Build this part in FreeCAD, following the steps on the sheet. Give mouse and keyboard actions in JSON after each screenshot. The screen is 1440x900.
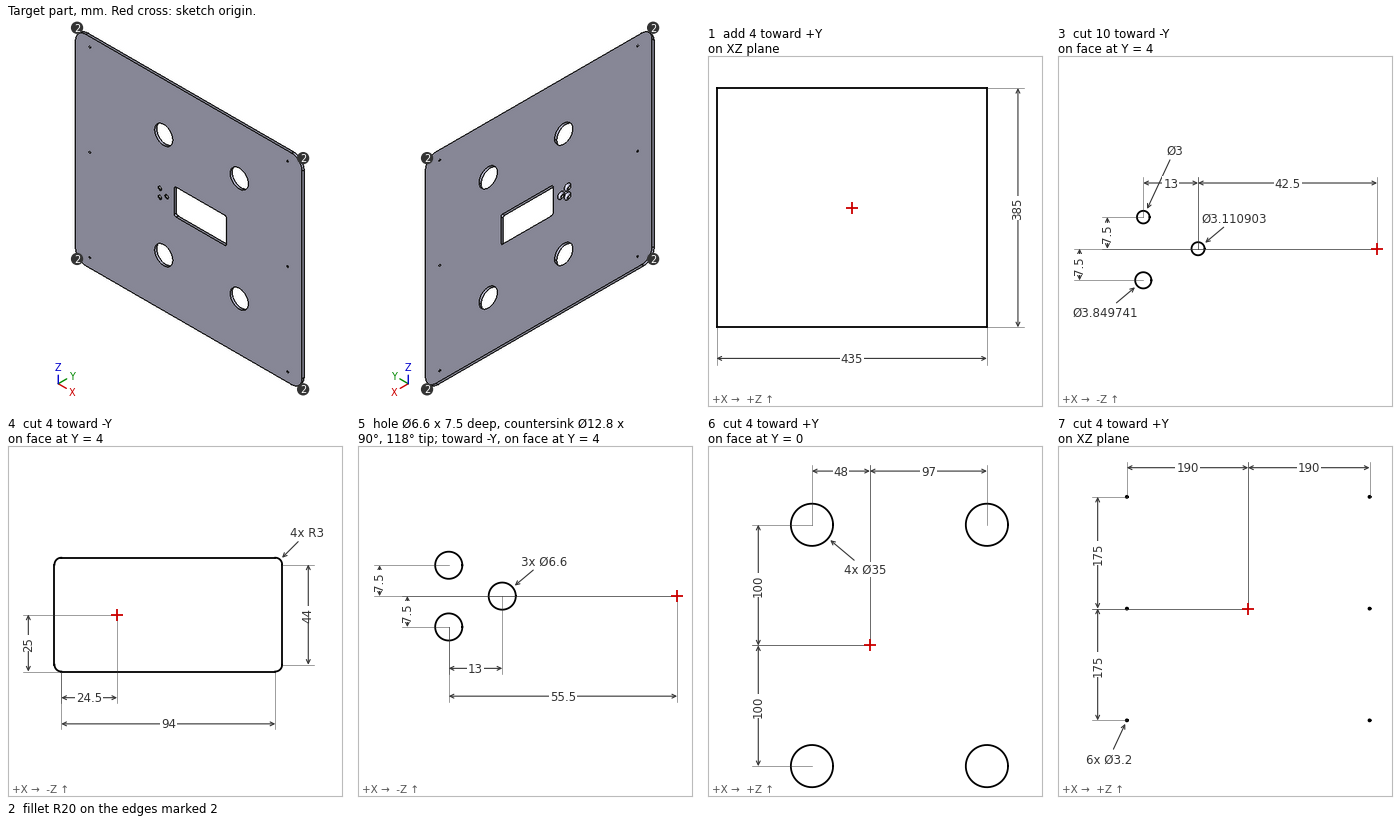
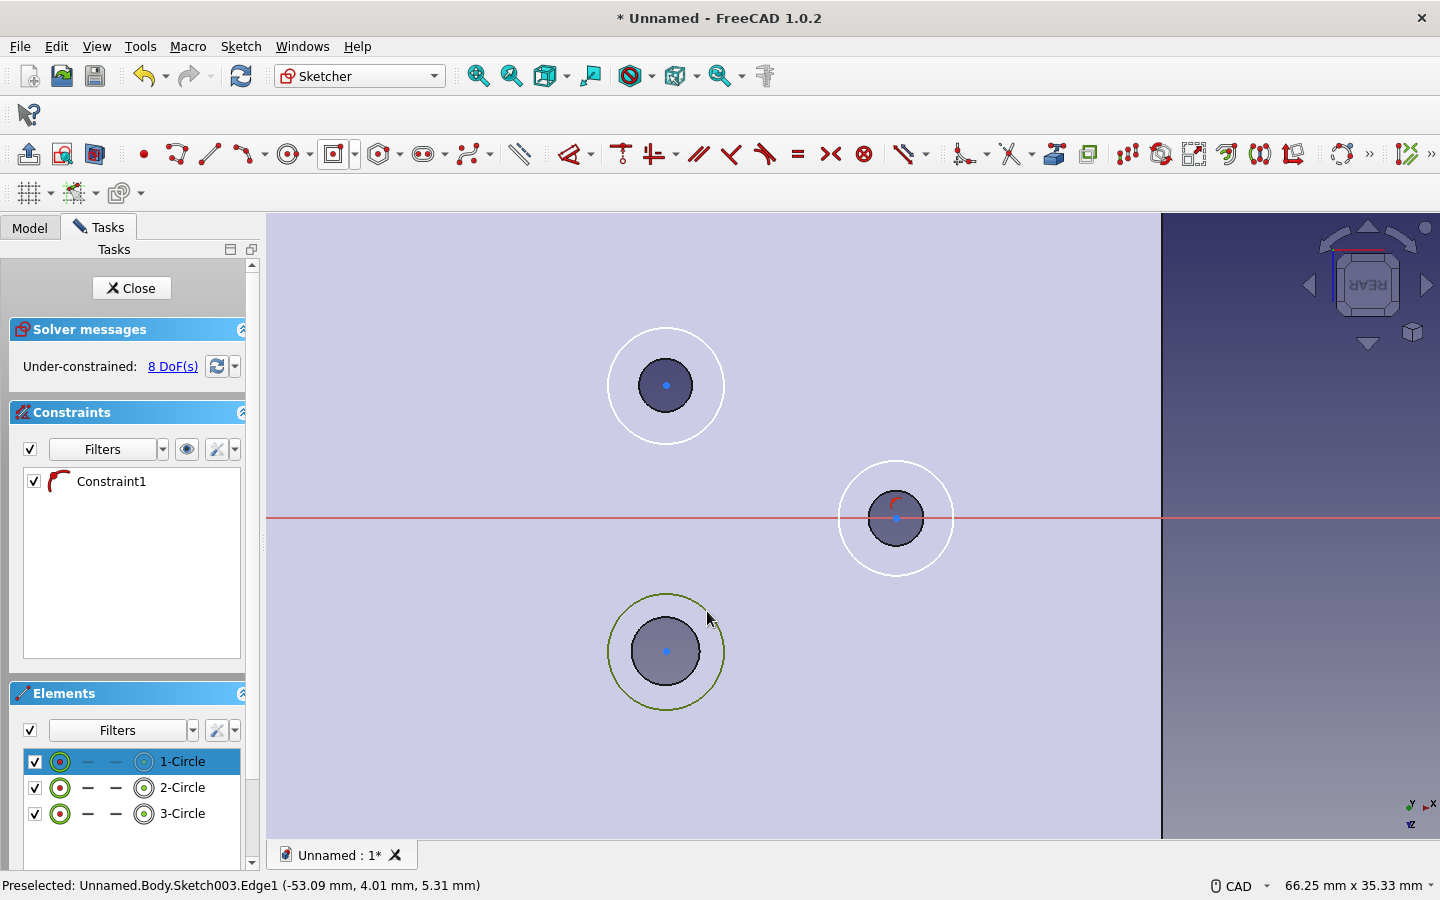
{"action": "left_click", "coordinate": [937, 478]}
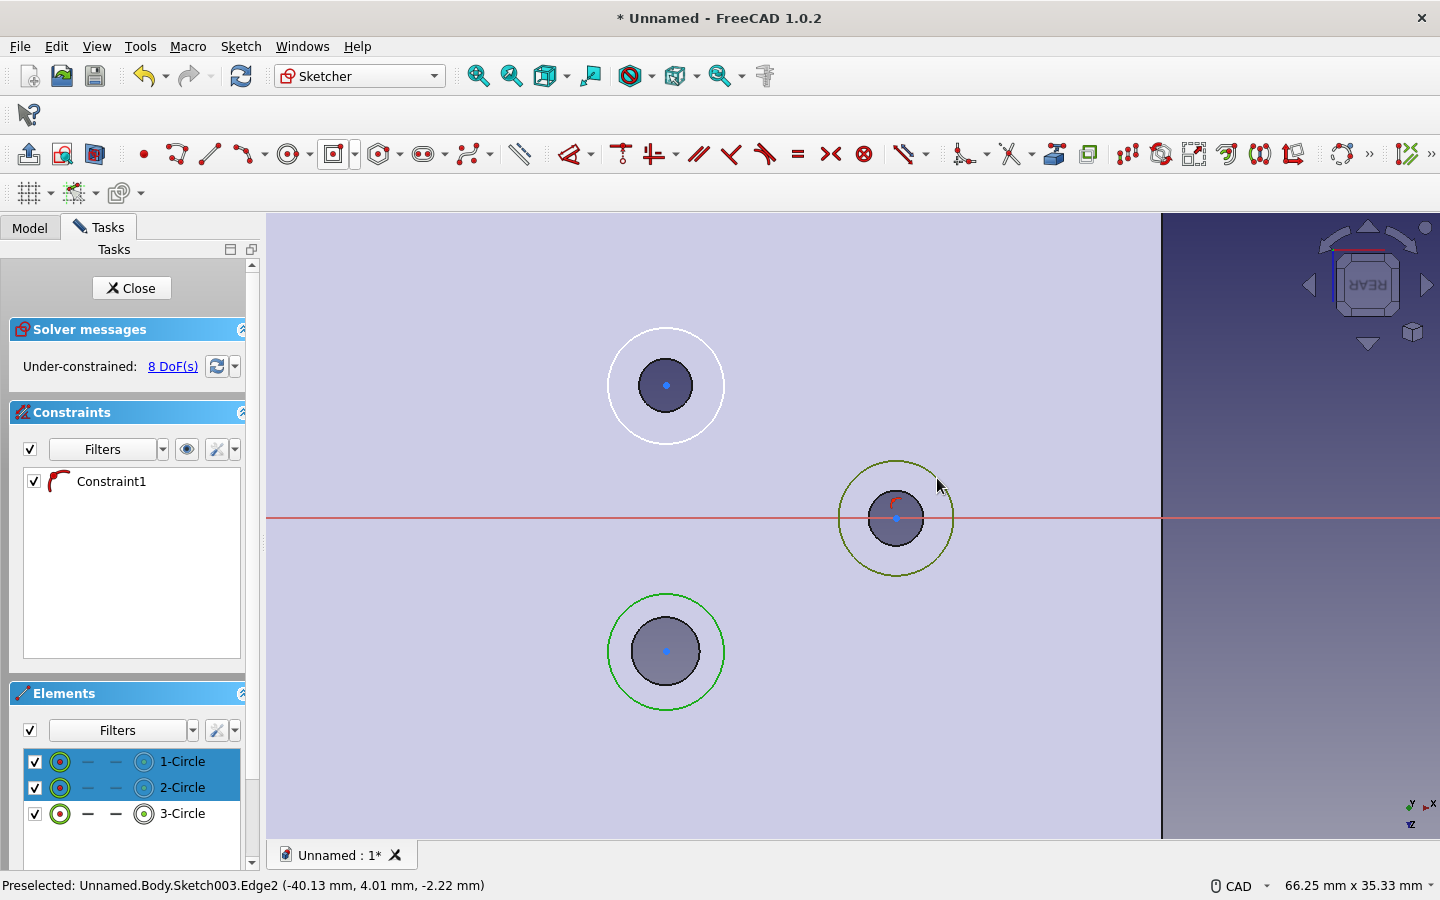
{"action": "left_click", "coordinate": [707, 345]}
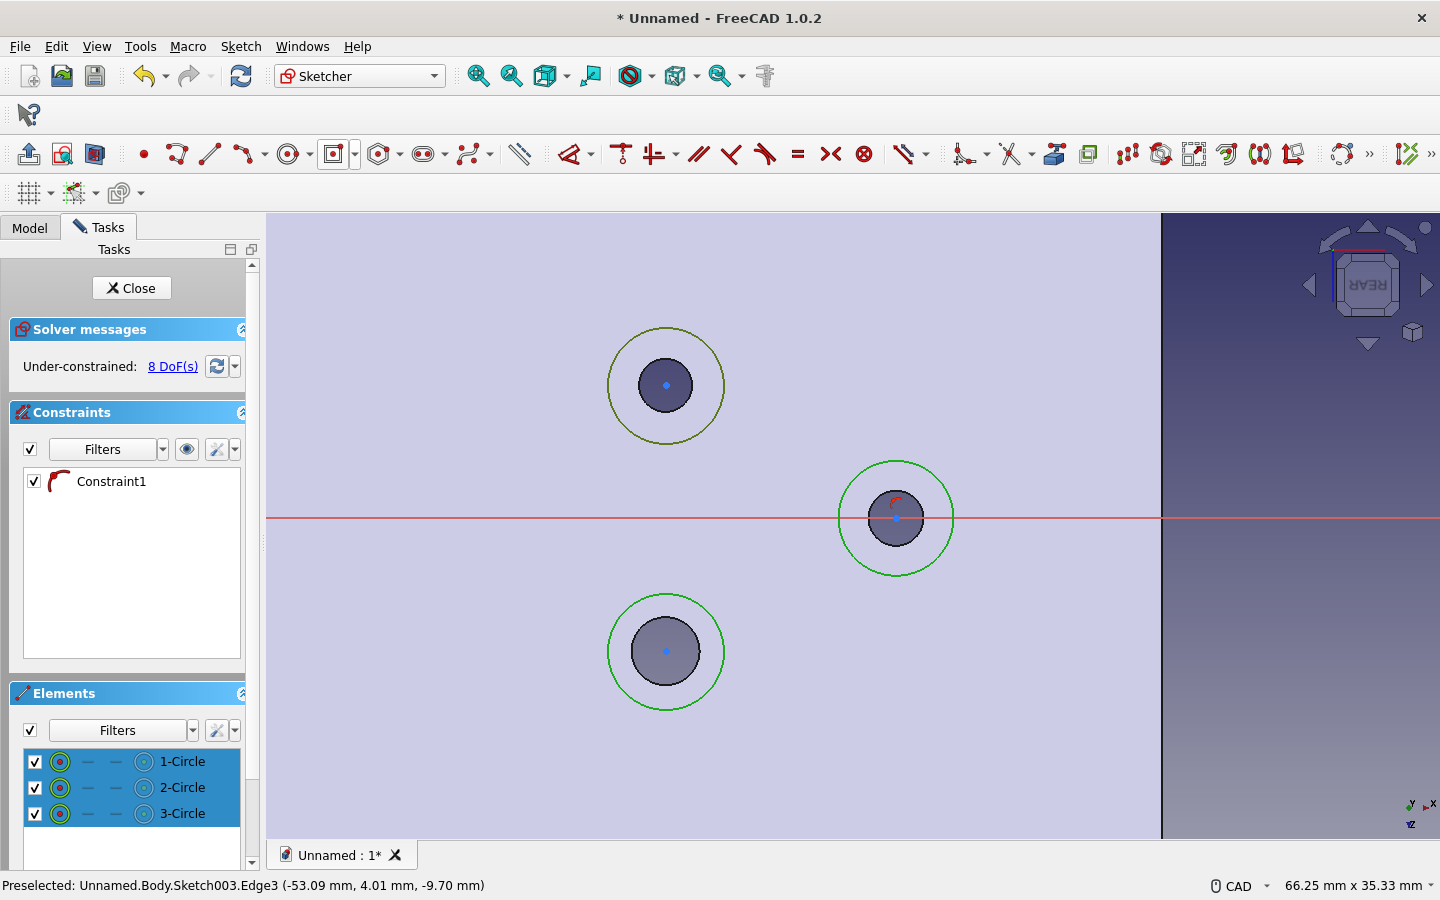
{"action": "left_click", "coordinate": [798, 154]}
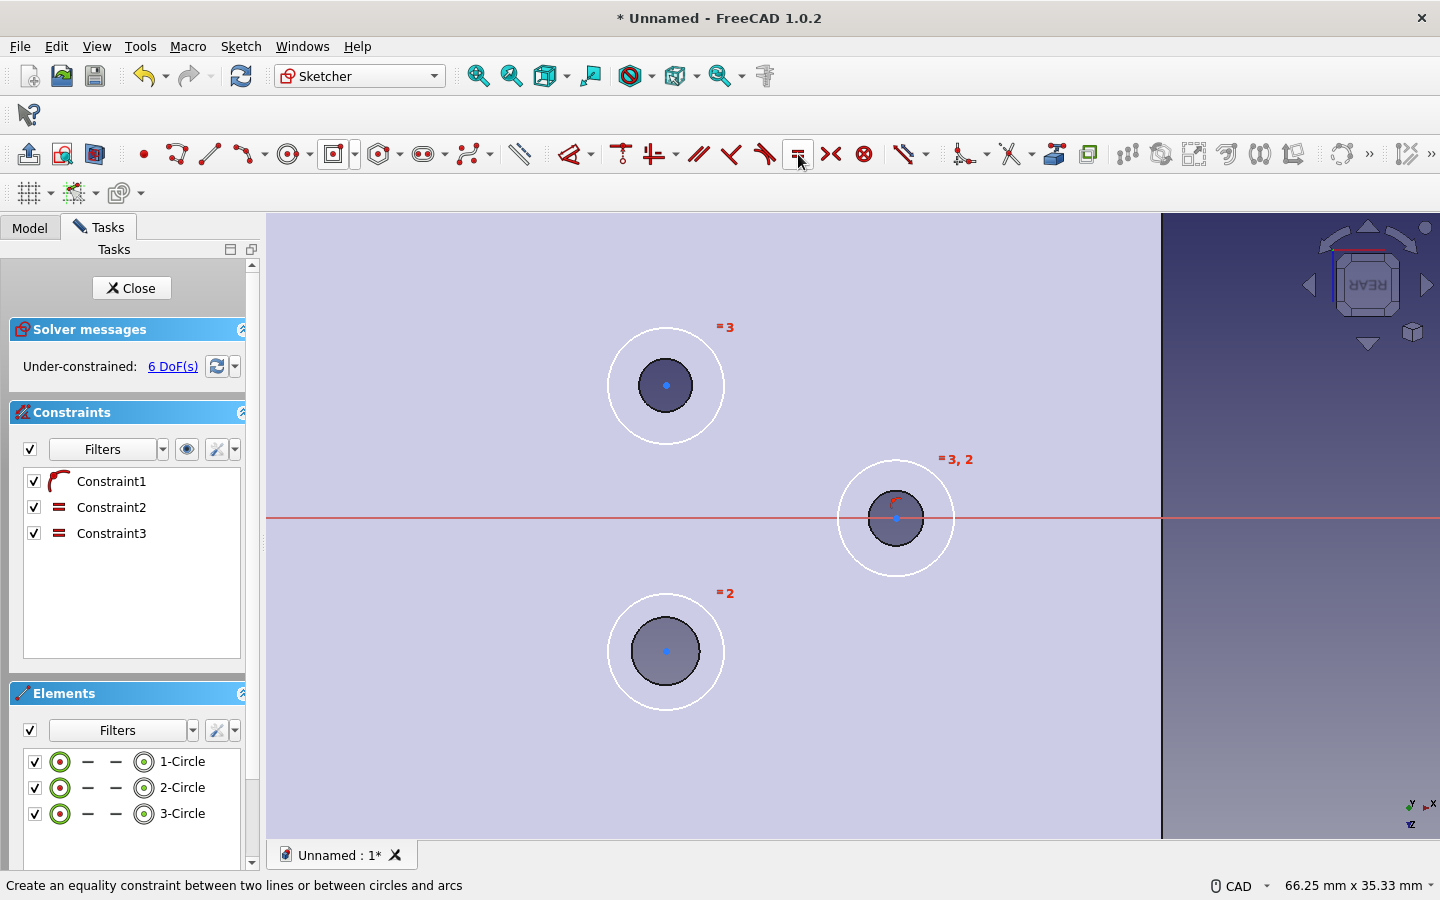
{"action": "left_click", "coordinate": [666, 652]}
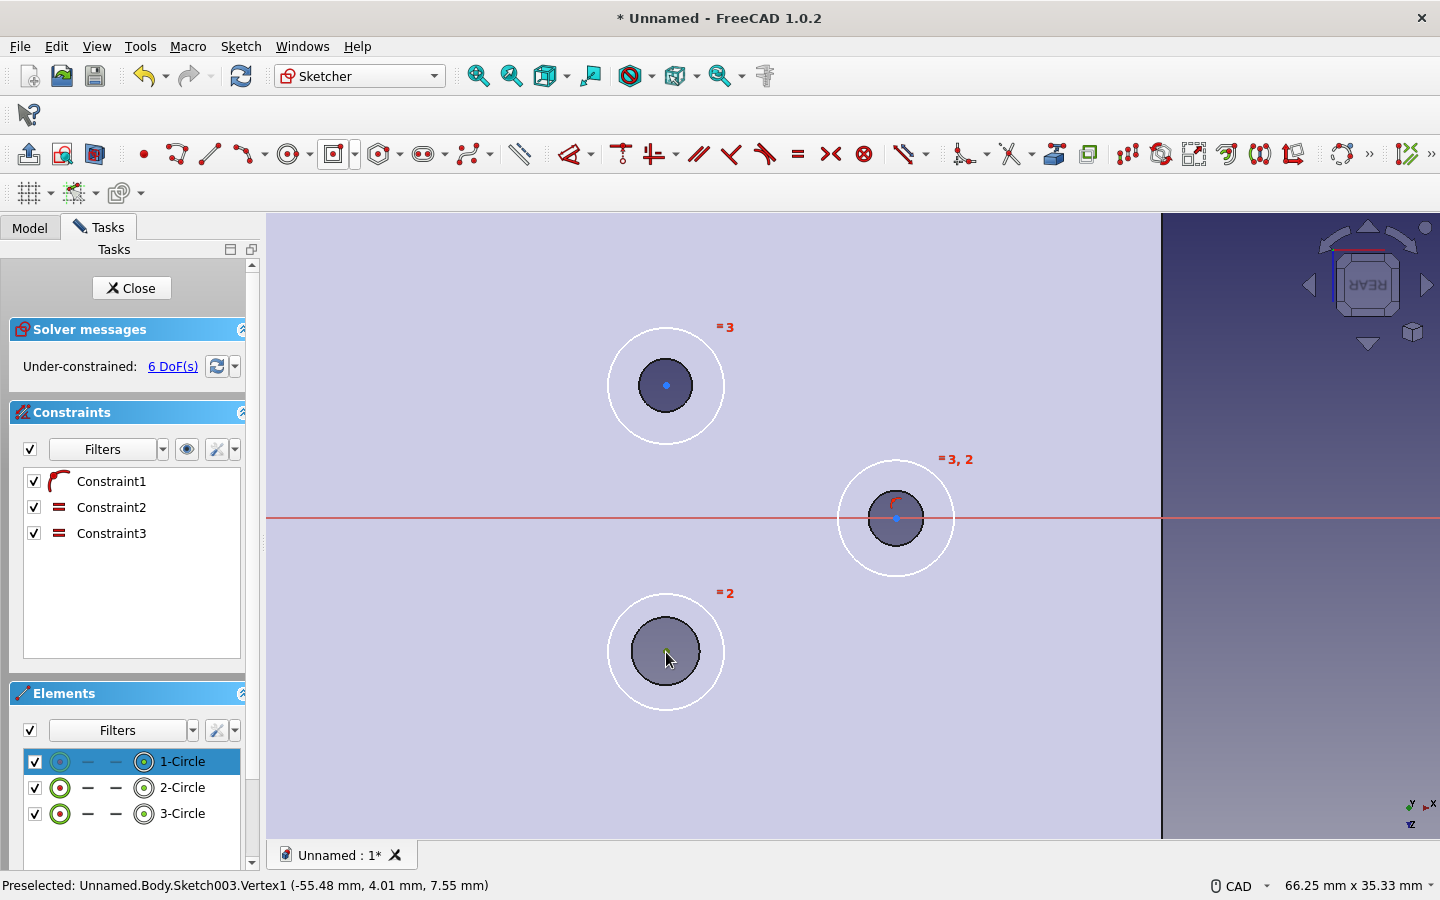
{"action": "left_click", "coordinate": [666, 386]}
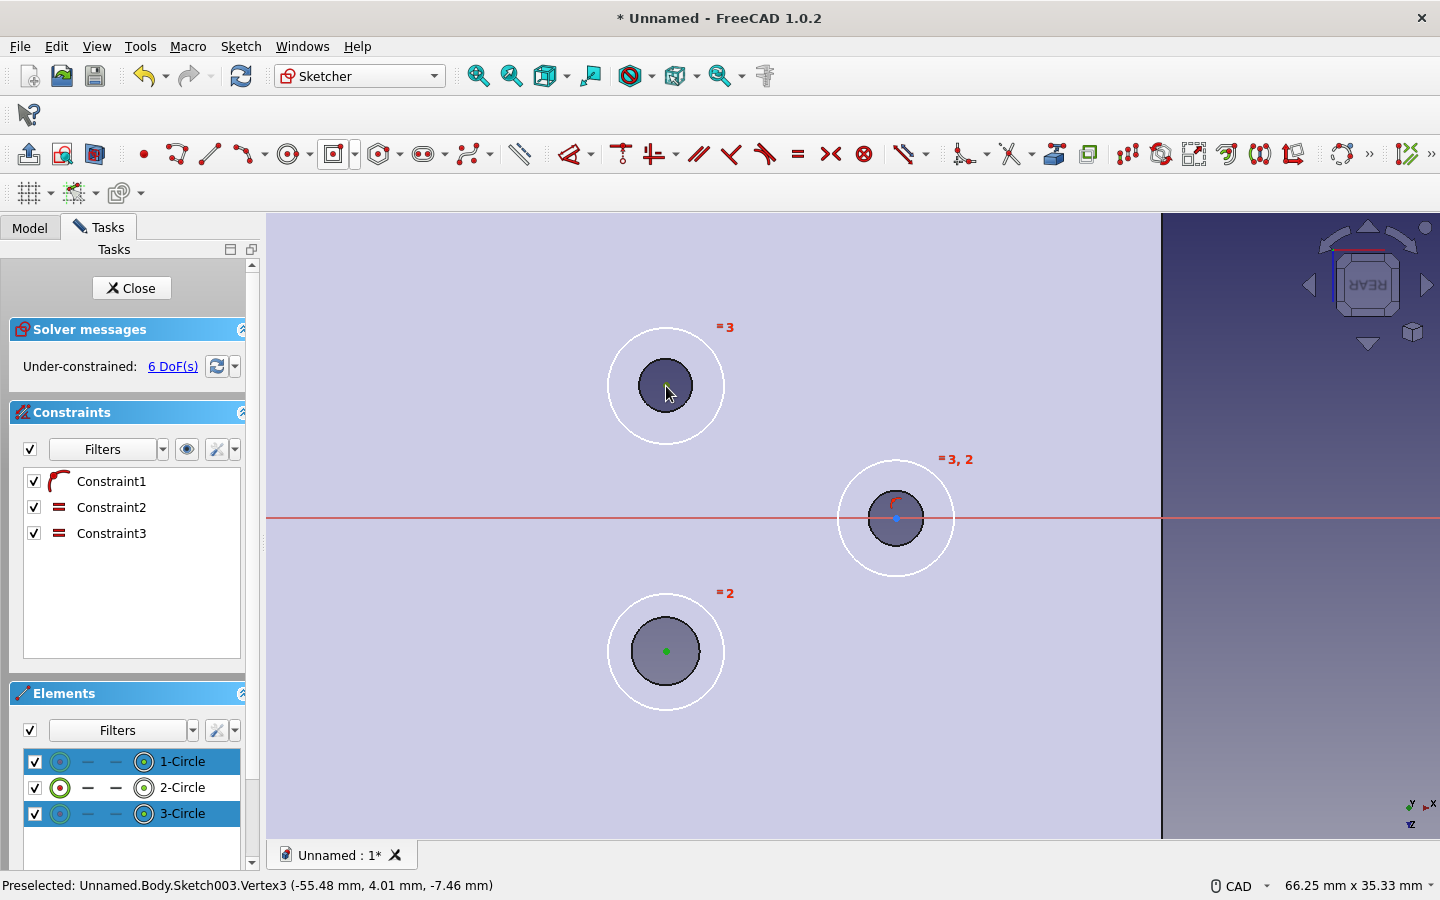
{"action": "key", "text": "v"}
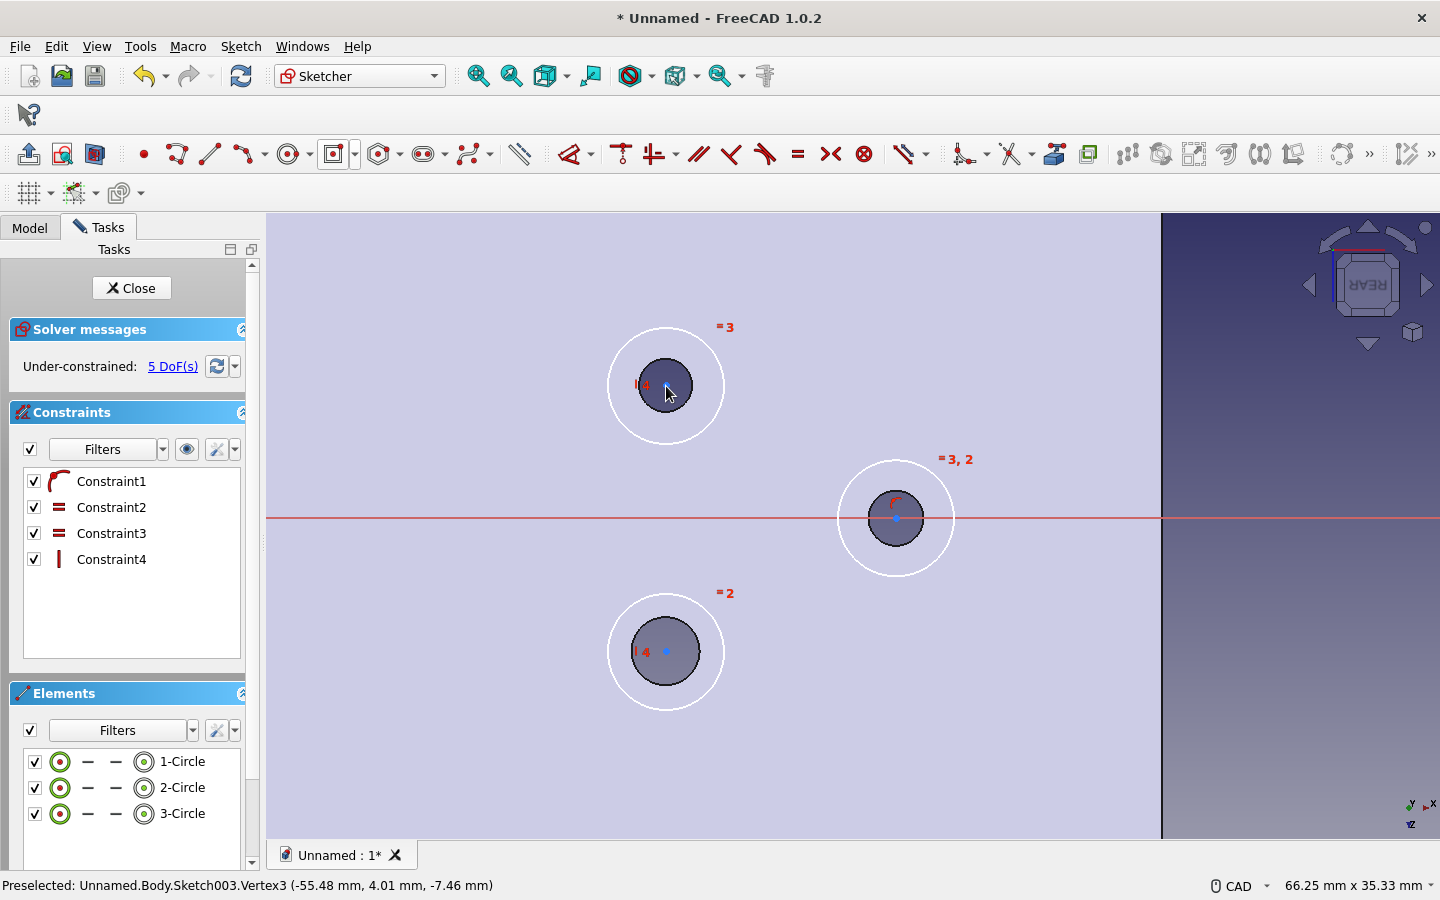
{"action": "left_click", "coordinate": [568, 154]}